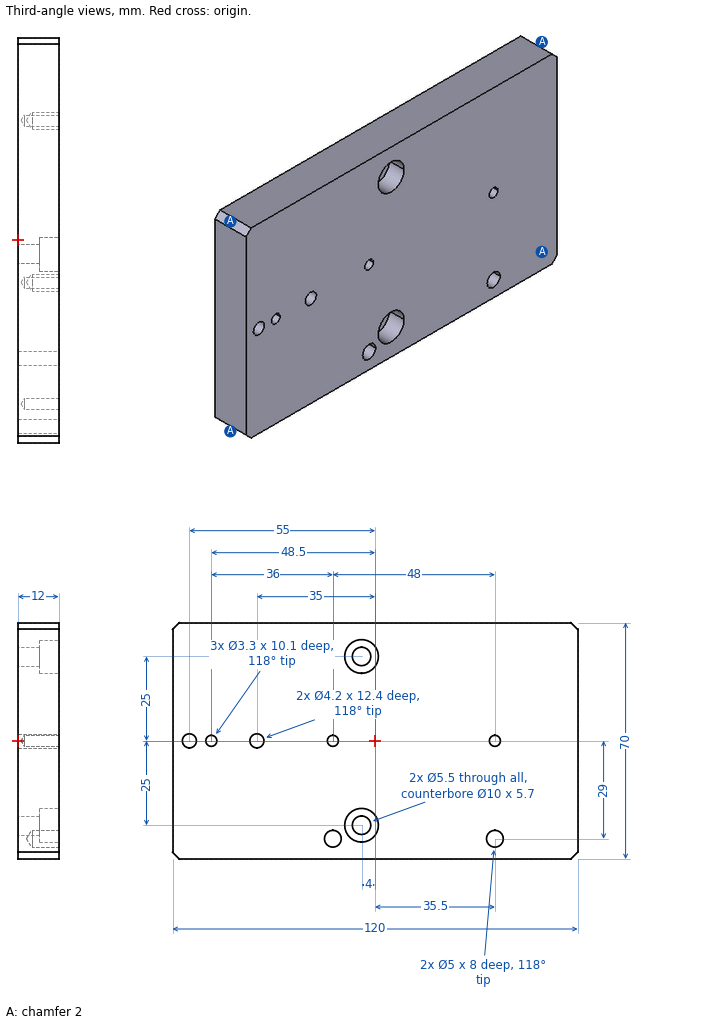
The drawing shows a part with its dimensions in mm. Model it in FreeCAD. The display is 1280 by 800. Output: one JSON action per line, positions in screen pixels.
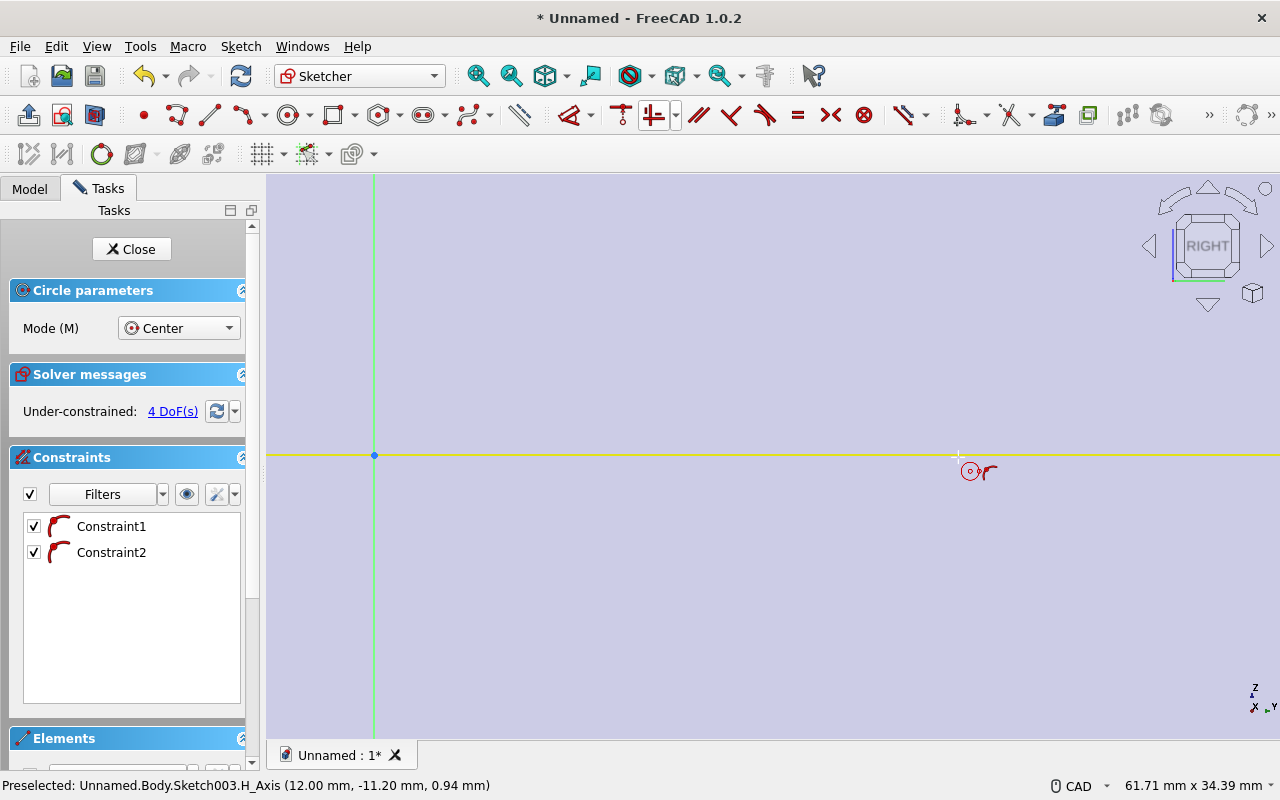
{"action": "left_click", "coordinate": [958, 455]}
{"action": "left_click", "coordinate": [977, 436]}
{"action": "key", "text": "Escape"}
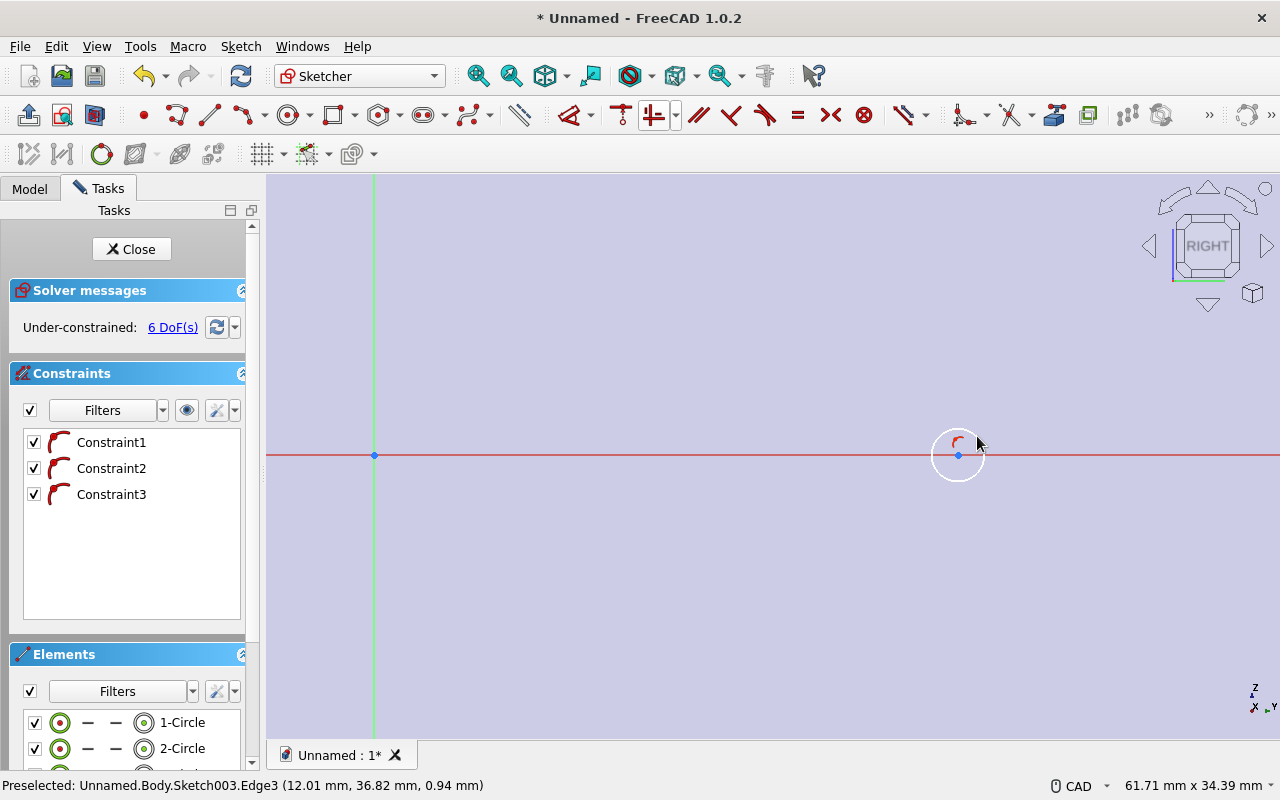
{"action": "scroll", "coordinate": [959, 457], "scroll_direction": "down", "scroll_amount": 5}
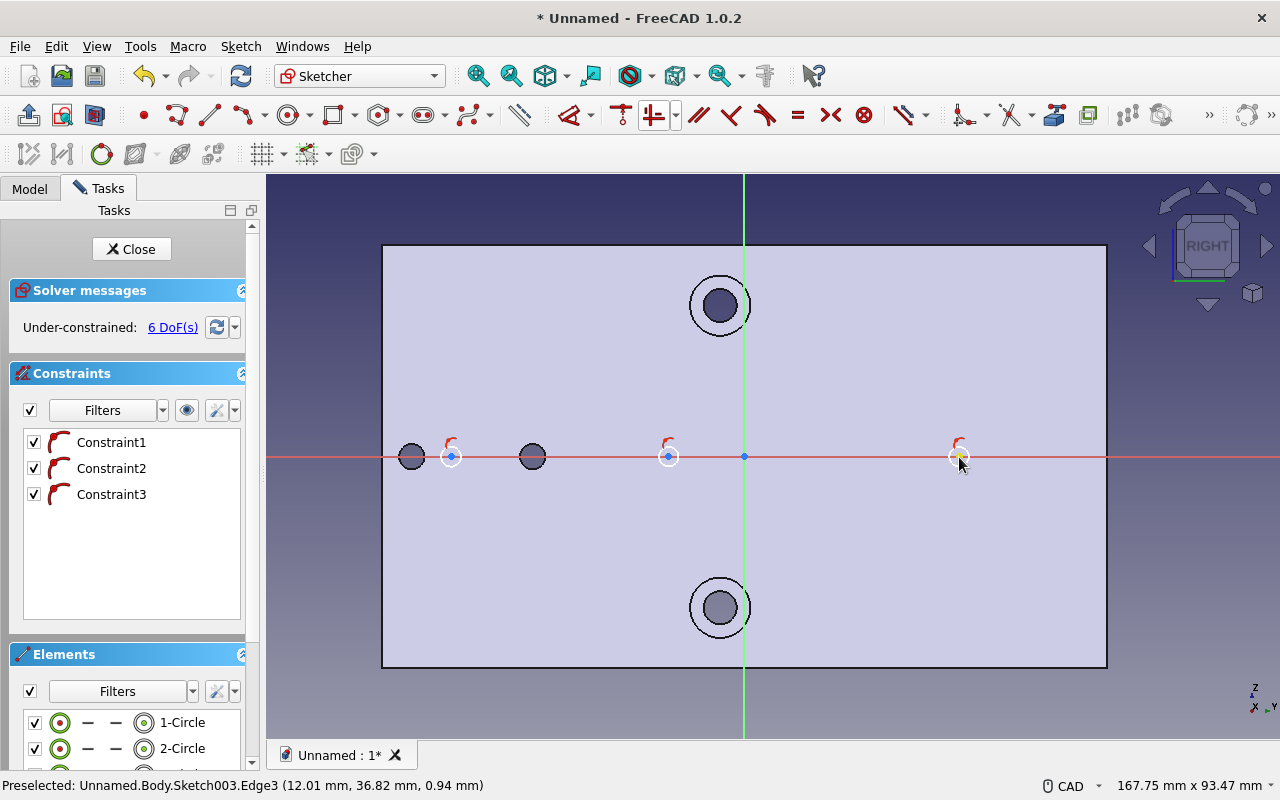
{"action": "scroll", "coordinate": [458, 450], "scroll_direction": "up", "scroll_amount": 4}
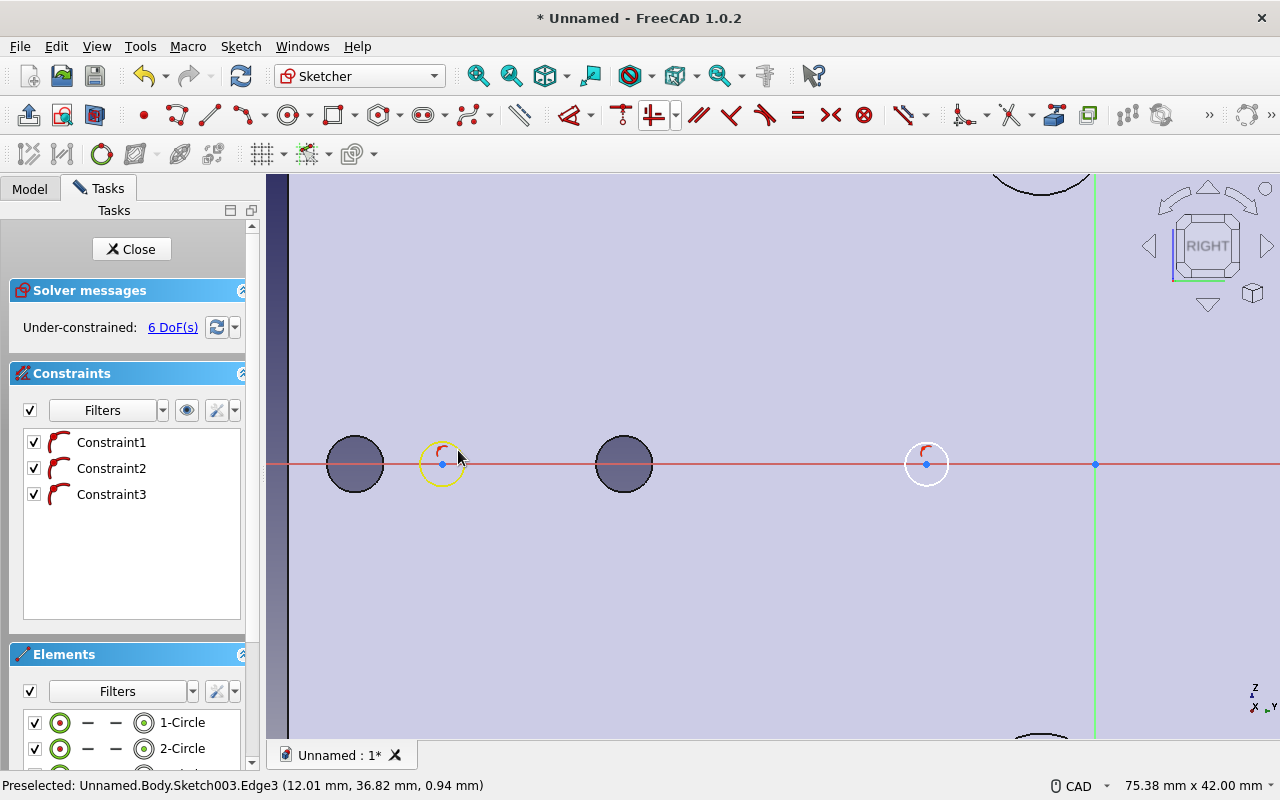
{"action": "left_click", "coordinate": [458, 448]}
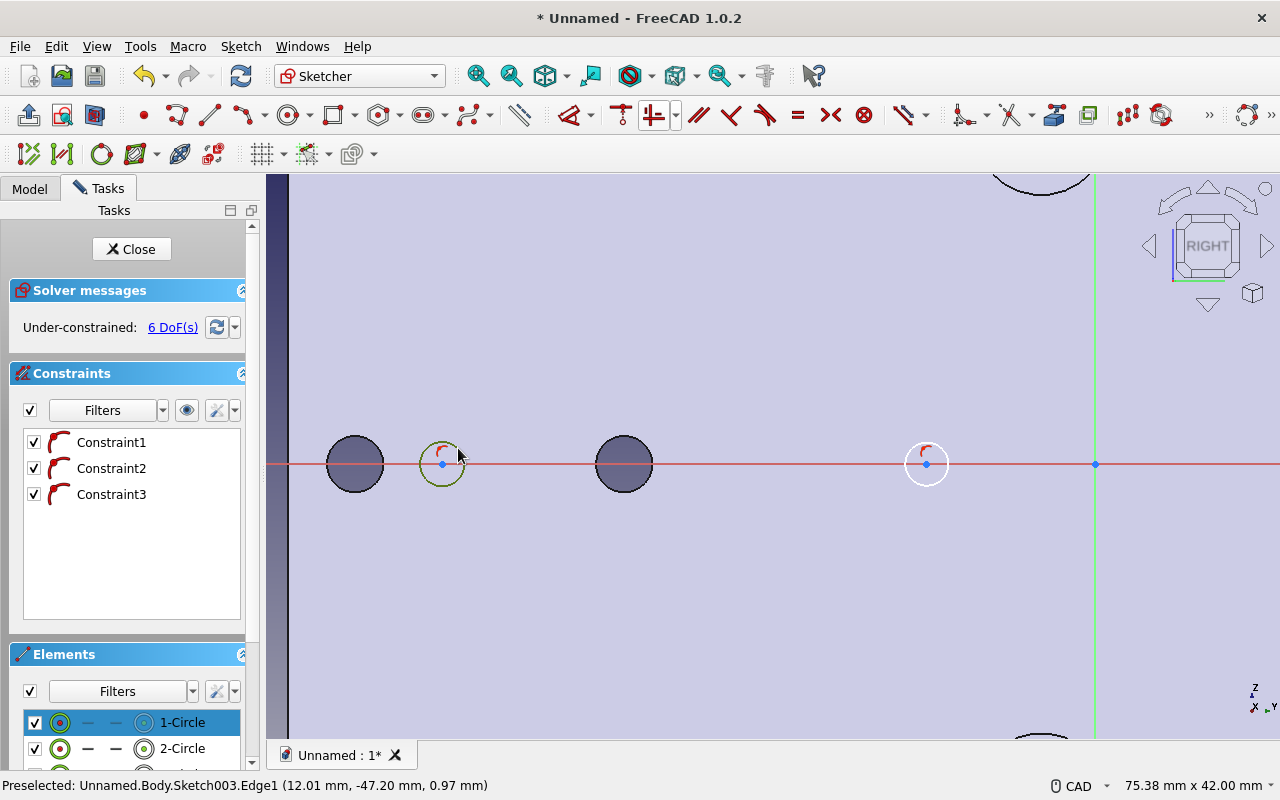
{"action": "left_click", "coordinate": [942, 449]}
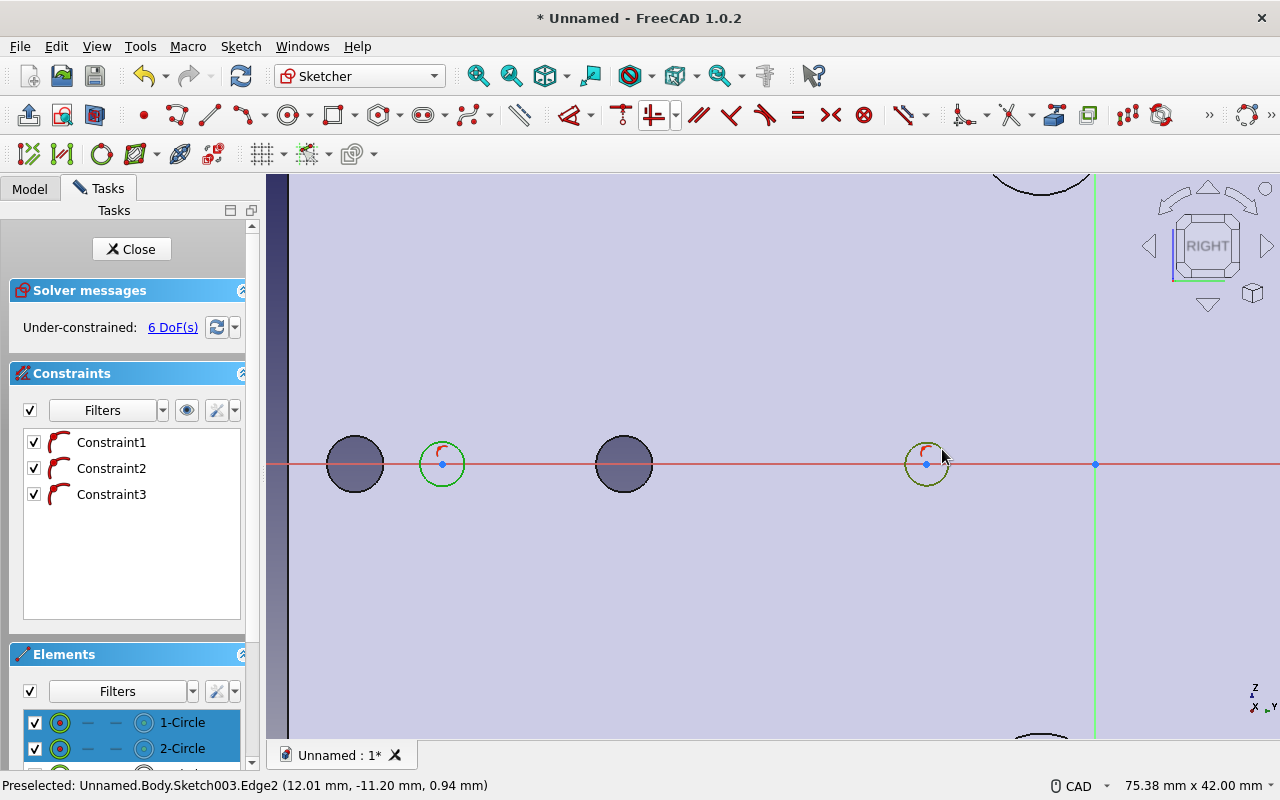
{"action": "scroll", "coordinate": [457, 450], "scroll_direction": "down", "scroll_amount": 4}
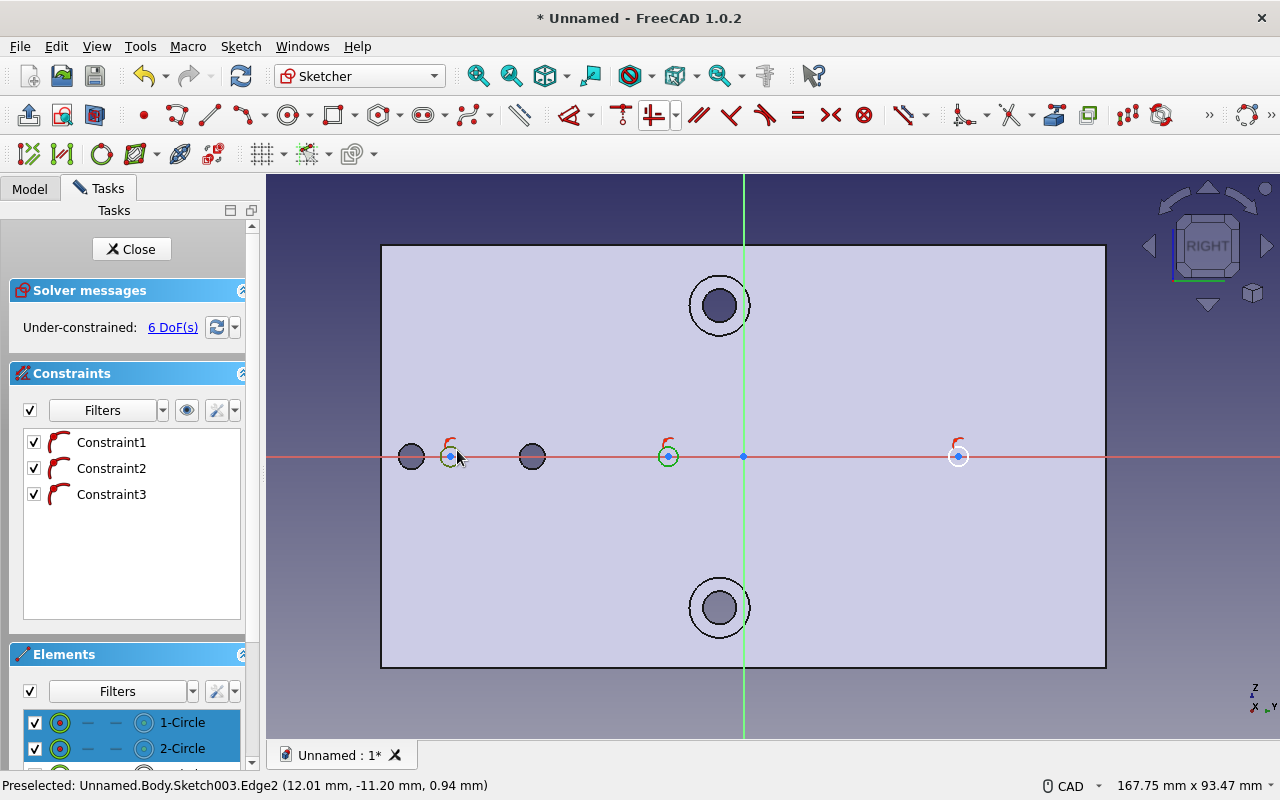
{"action": "scroll", "coordinate": [965, 450], "scroll_direction": "up", "scroll_amount": 4}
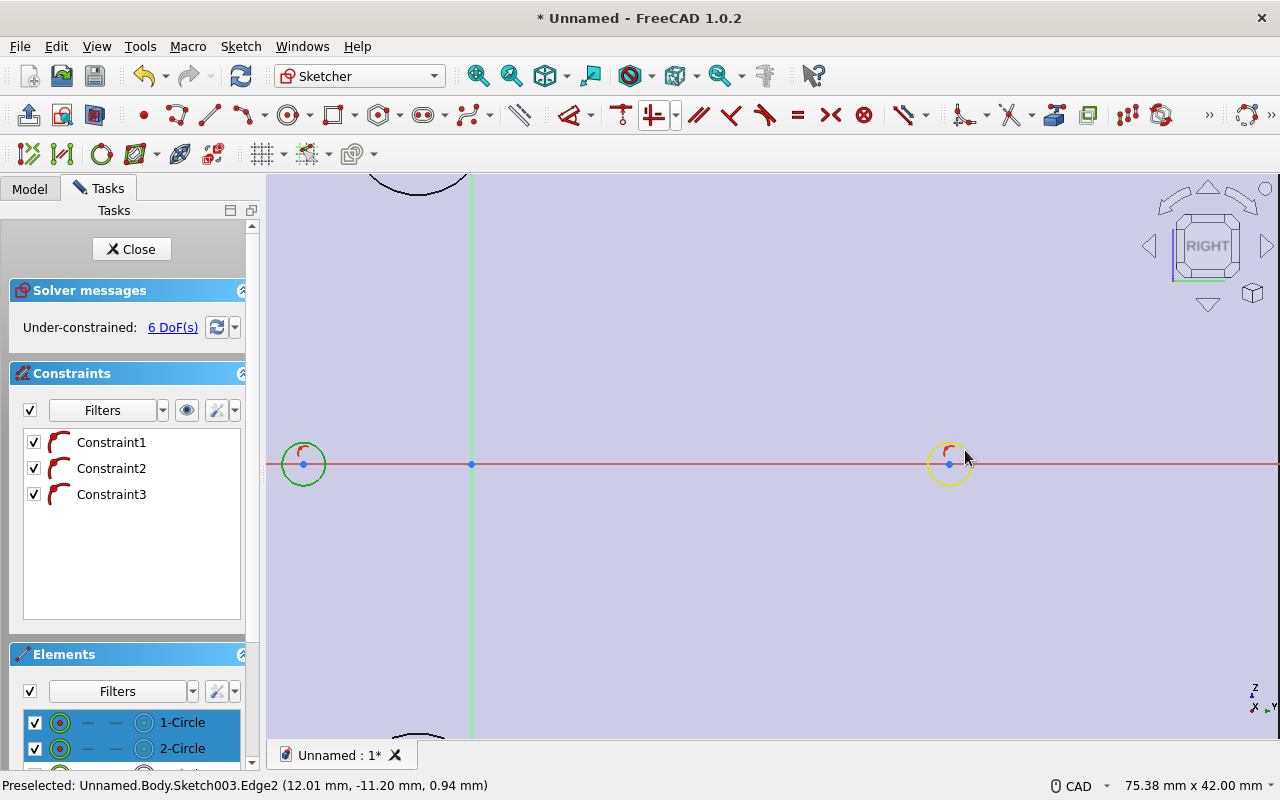
{"action": "left_click", "coordinate": [965, 449]}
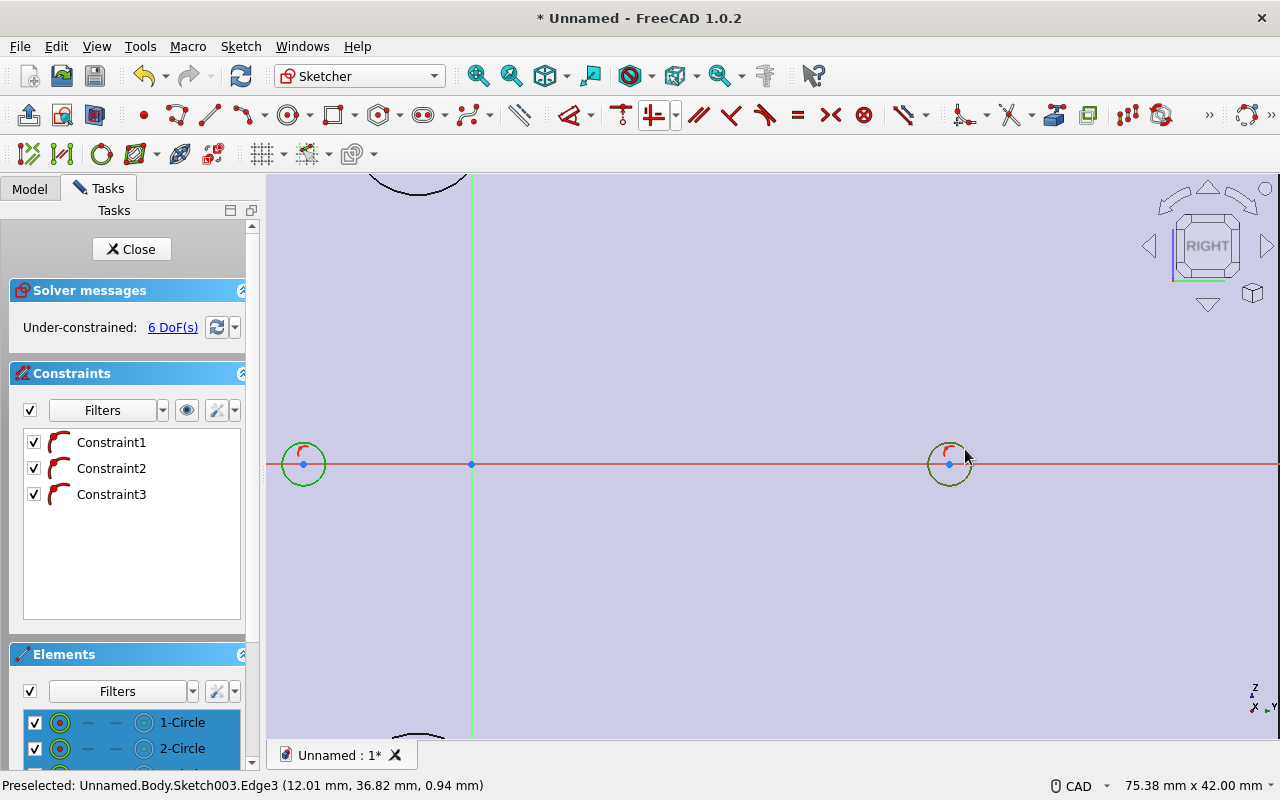
{"action": "left_click", "coordinate": [798, 116]}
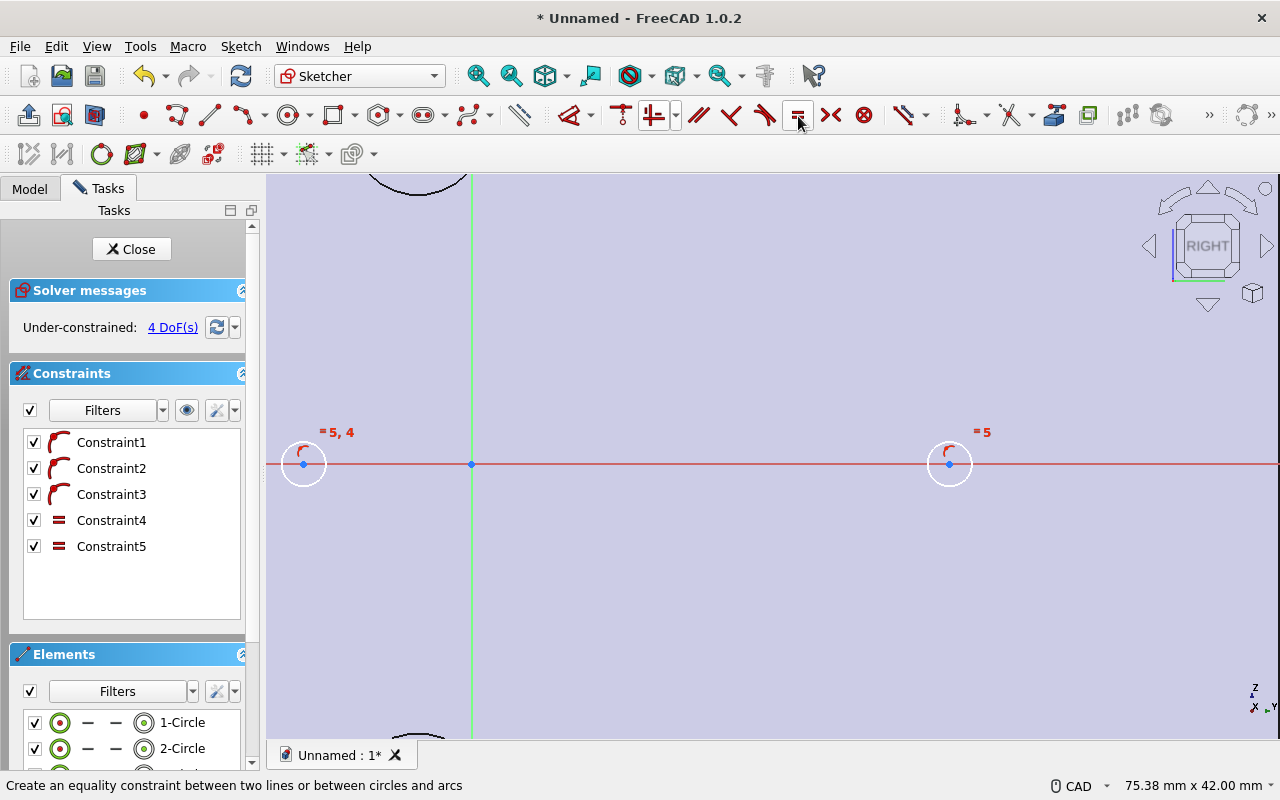
{"action": "left_click", "coordinate": [568, 116]}